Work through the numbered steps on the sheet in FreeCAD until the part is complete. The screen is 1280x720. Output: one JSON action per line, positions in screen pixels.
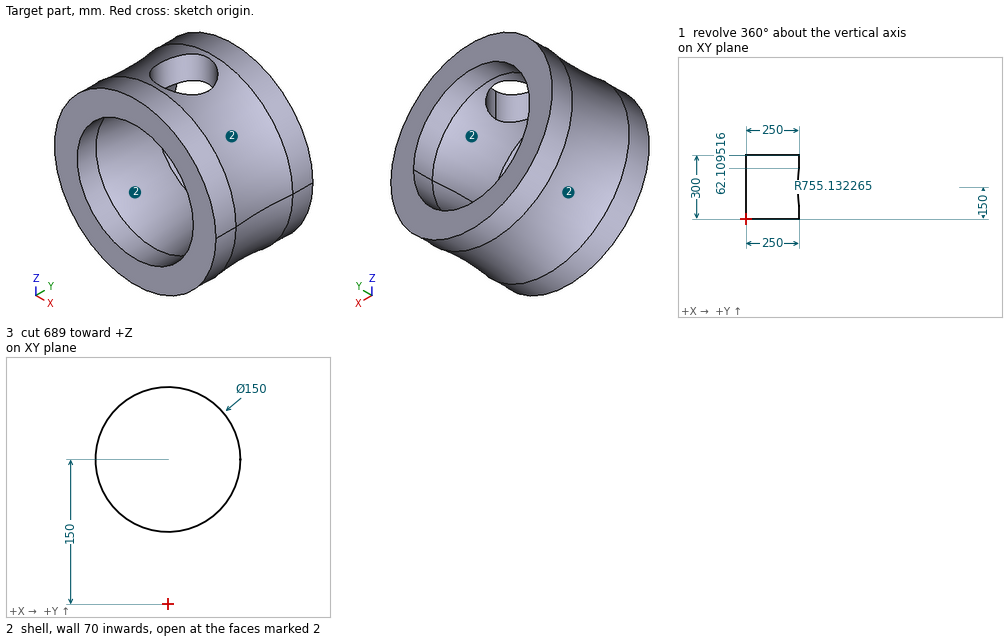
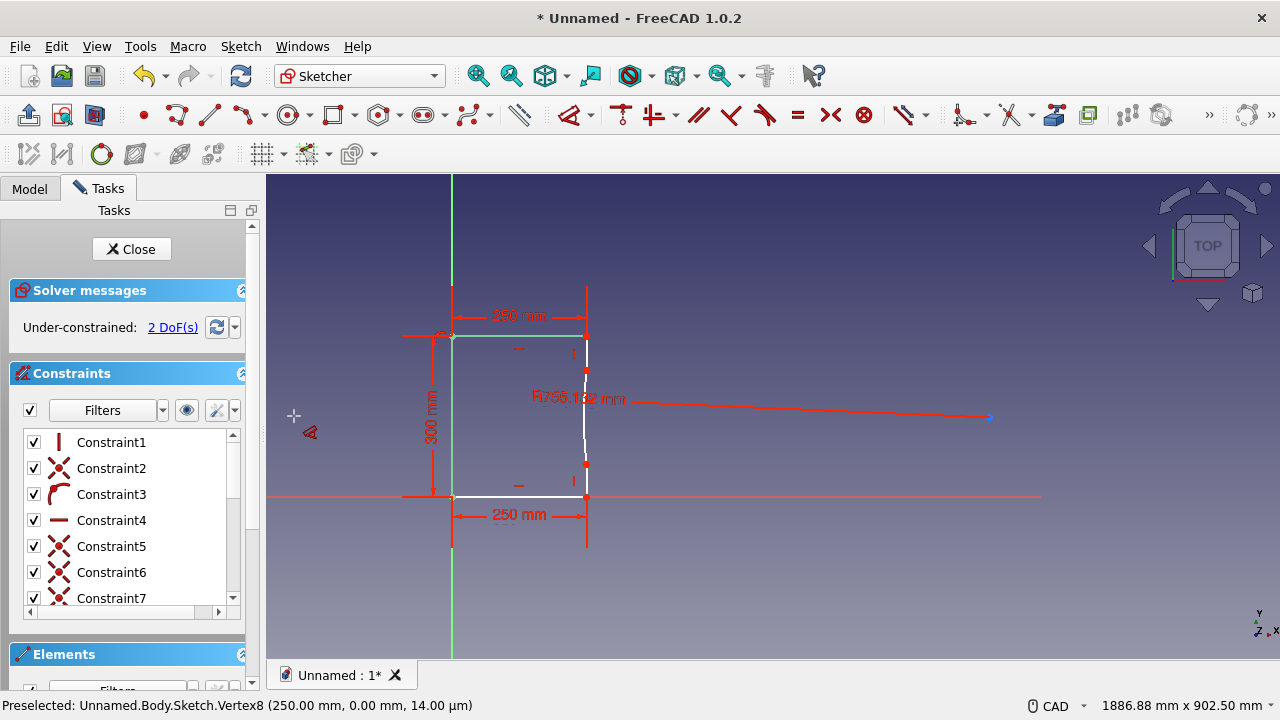
{"action": "left_click", "coordinate": [990, 417]}
{"action": "left_click", "coordinate": [1024, 457]}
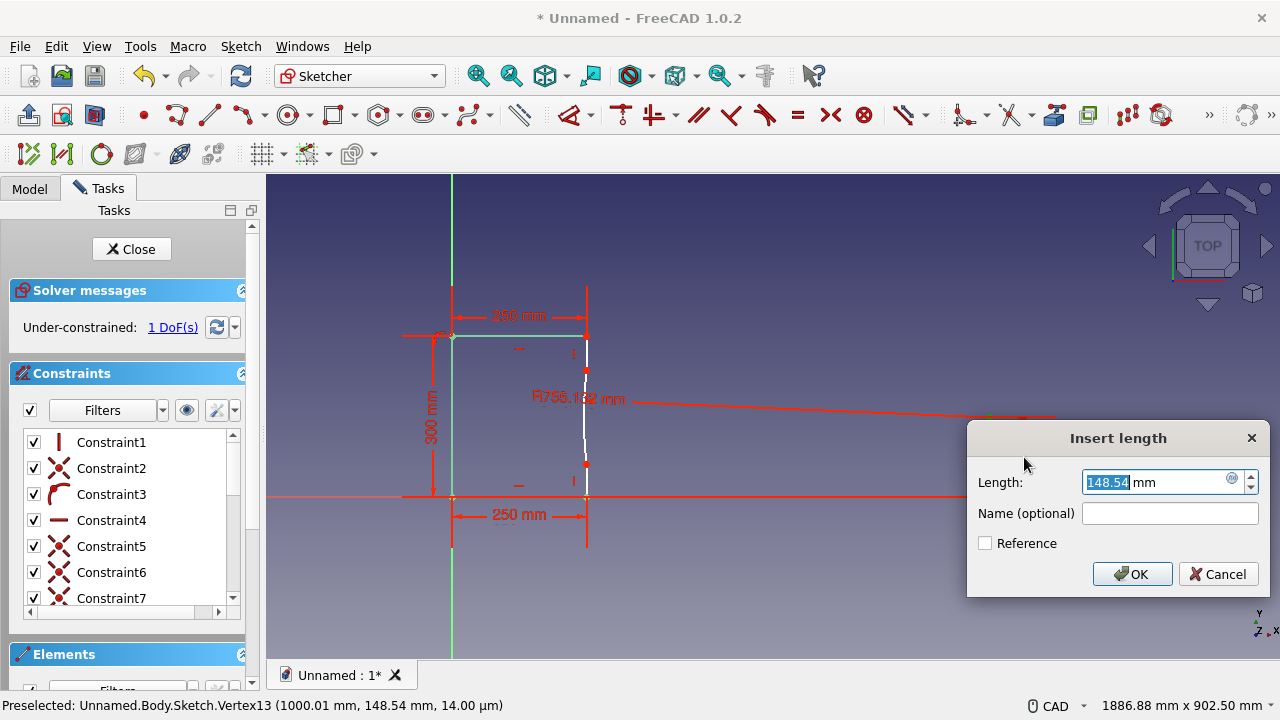
{"action": "type", "text": "150"}
{"action": "key", "text": "Return"}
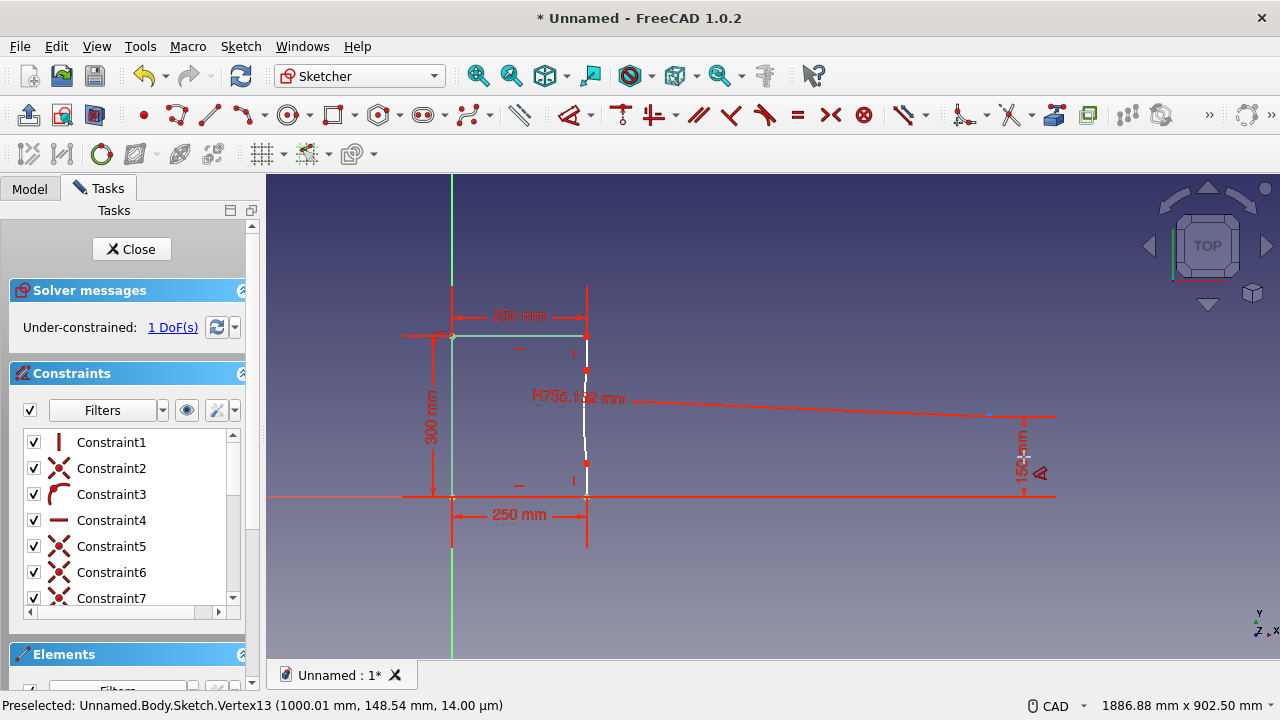
{"action": "scroll", "coordinate": [587, 360], "scroll_direction": "up", "scroll_amount": 2}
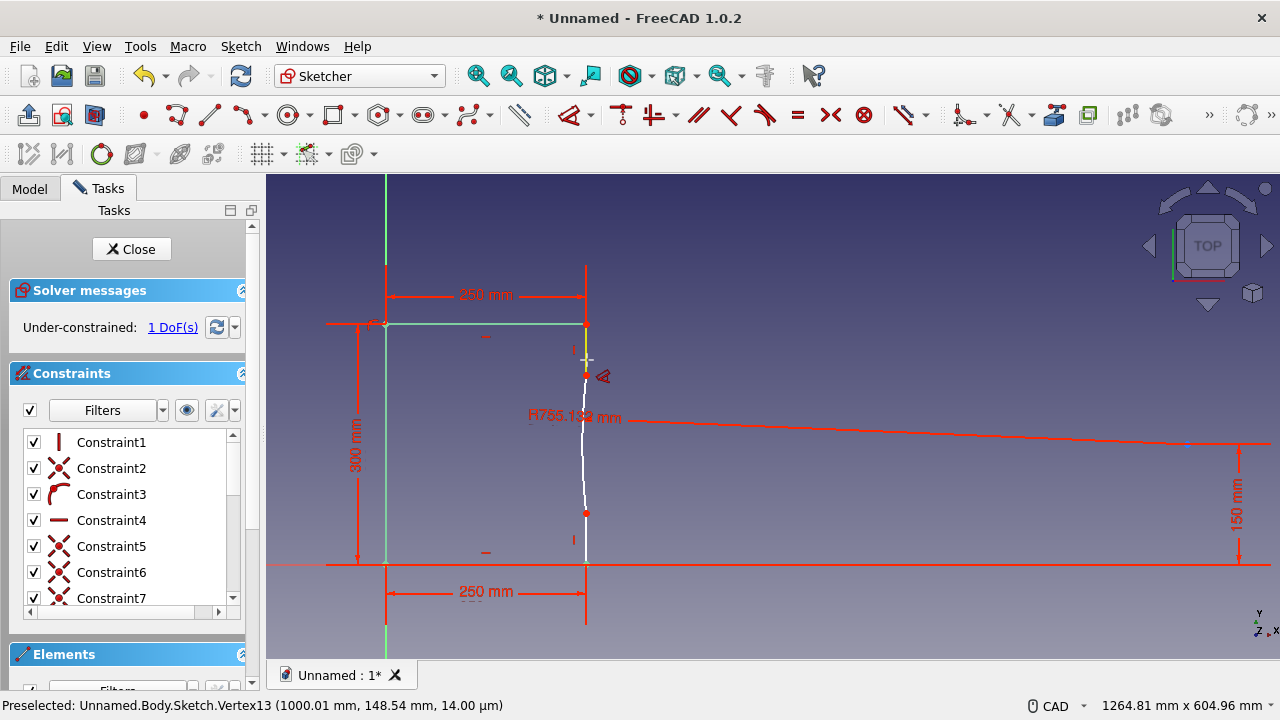
{"action": "left_click", "coordinate": [586, 360]}
{"action": "left_click", "coordinate": [620, 350]}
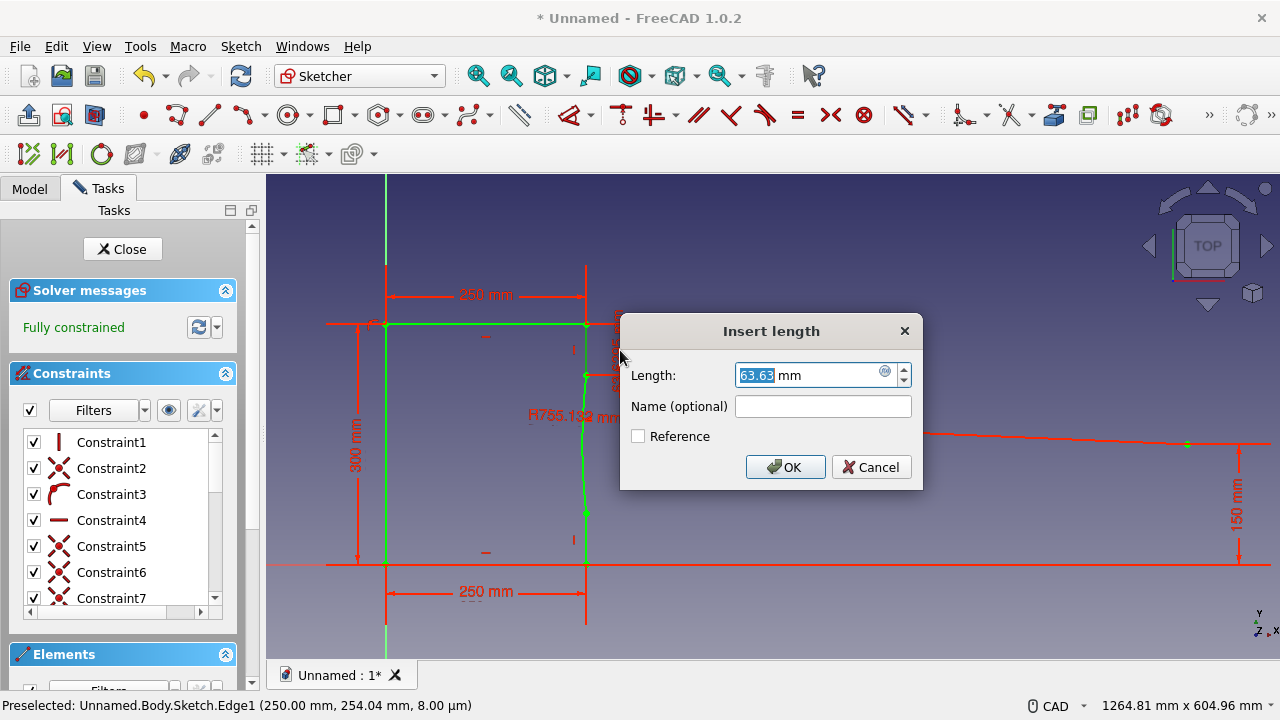
{"action": "type", "text": "62.109516"}
{"action": "key", "text": "Return"}
{"action": "key", "text": "Escape"}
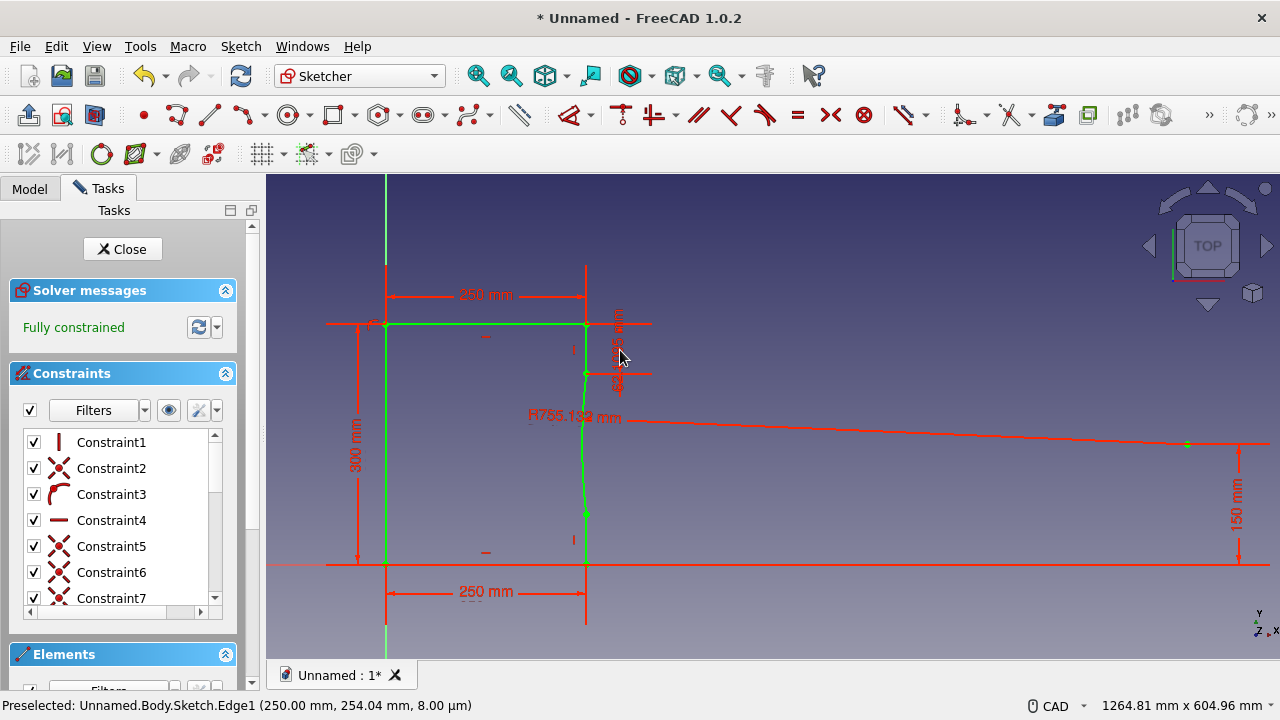
{"action": "left_click", "coordinate": [123, 249]}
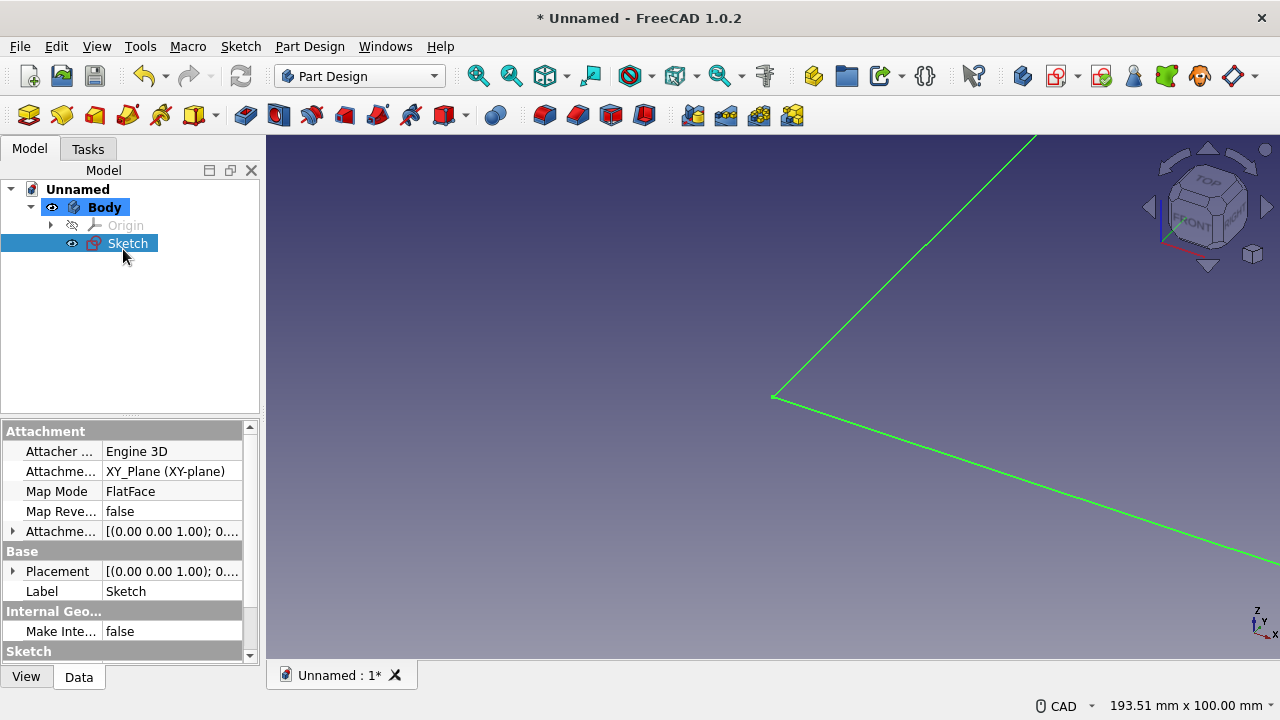
{"action": "left_click", "coordinate": [62, 116]}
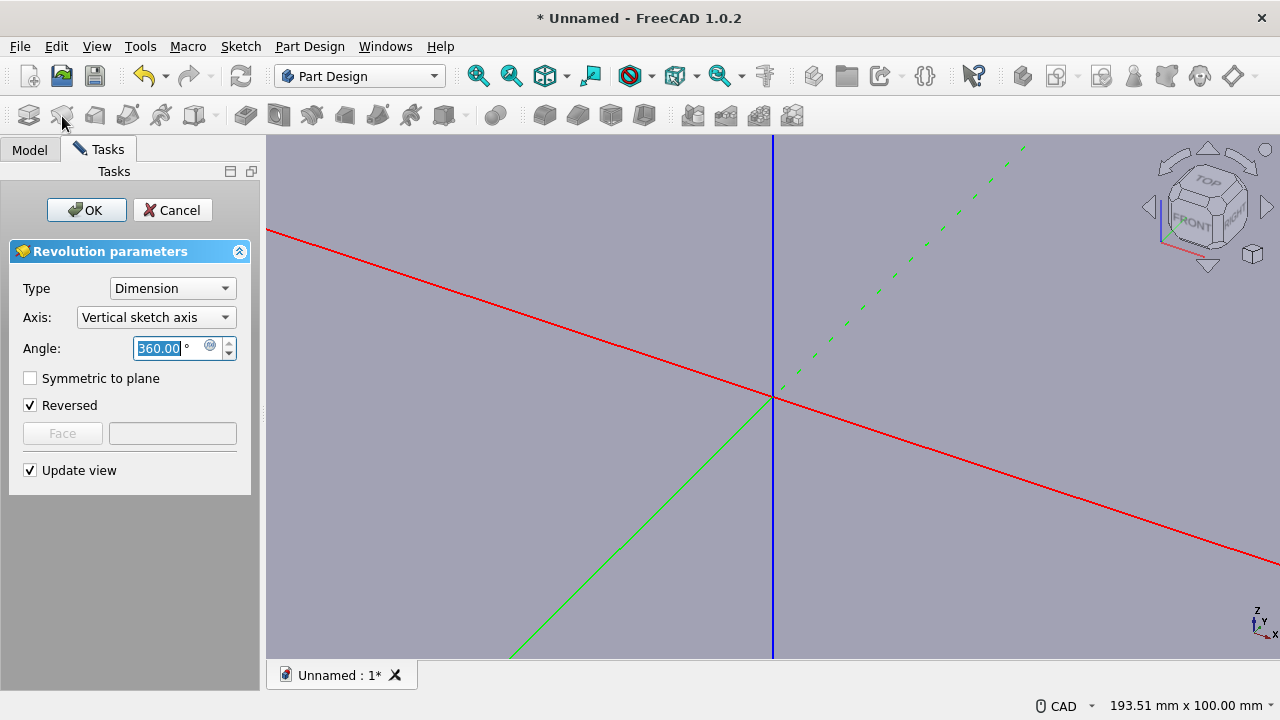
{"action": "left_click", "coordinate": [87, 210]}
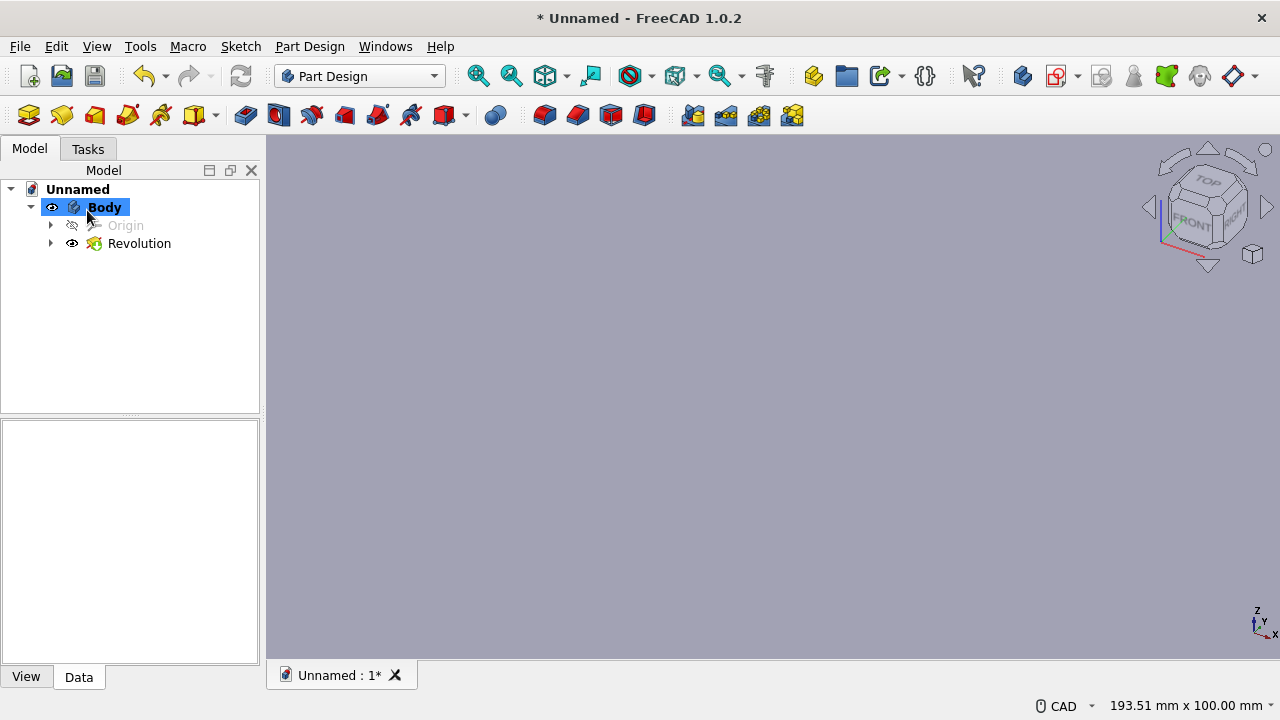
{"action": "left_click", "coordinate": [479, 76]}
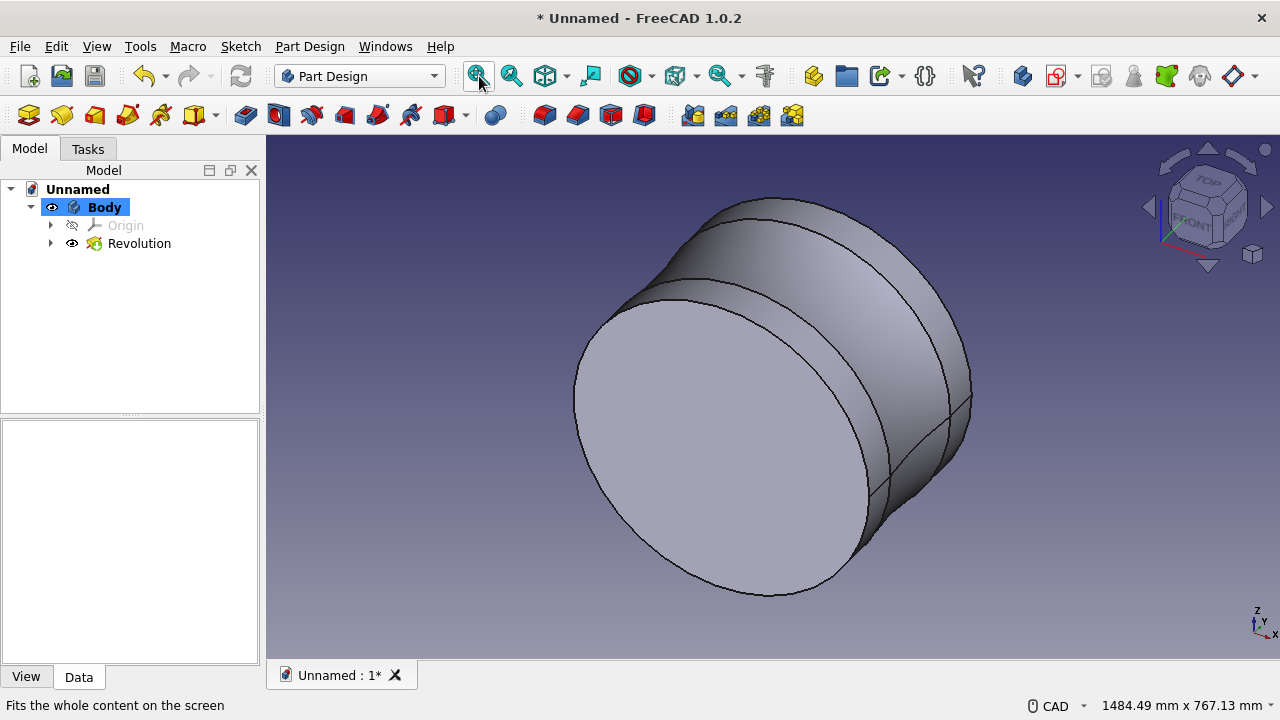
{"action": "left_click", "coordinate": [721, 447]}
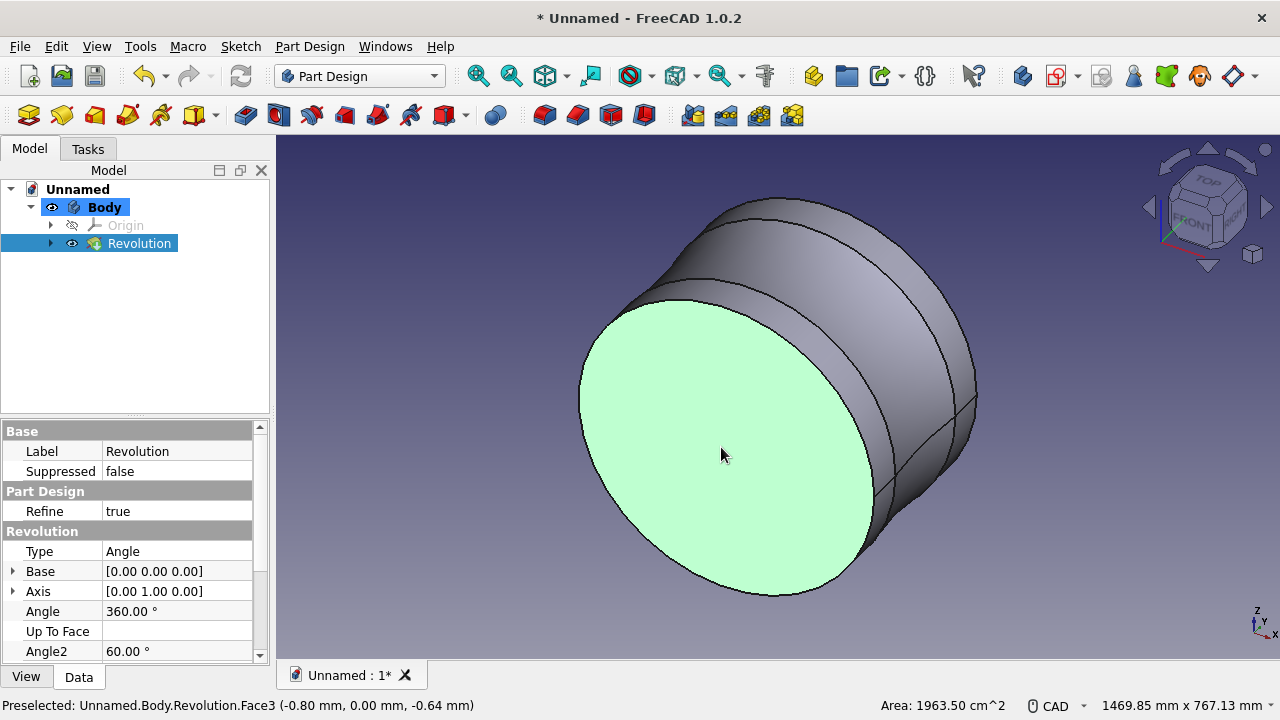
{"action": "key", "text": "0"}